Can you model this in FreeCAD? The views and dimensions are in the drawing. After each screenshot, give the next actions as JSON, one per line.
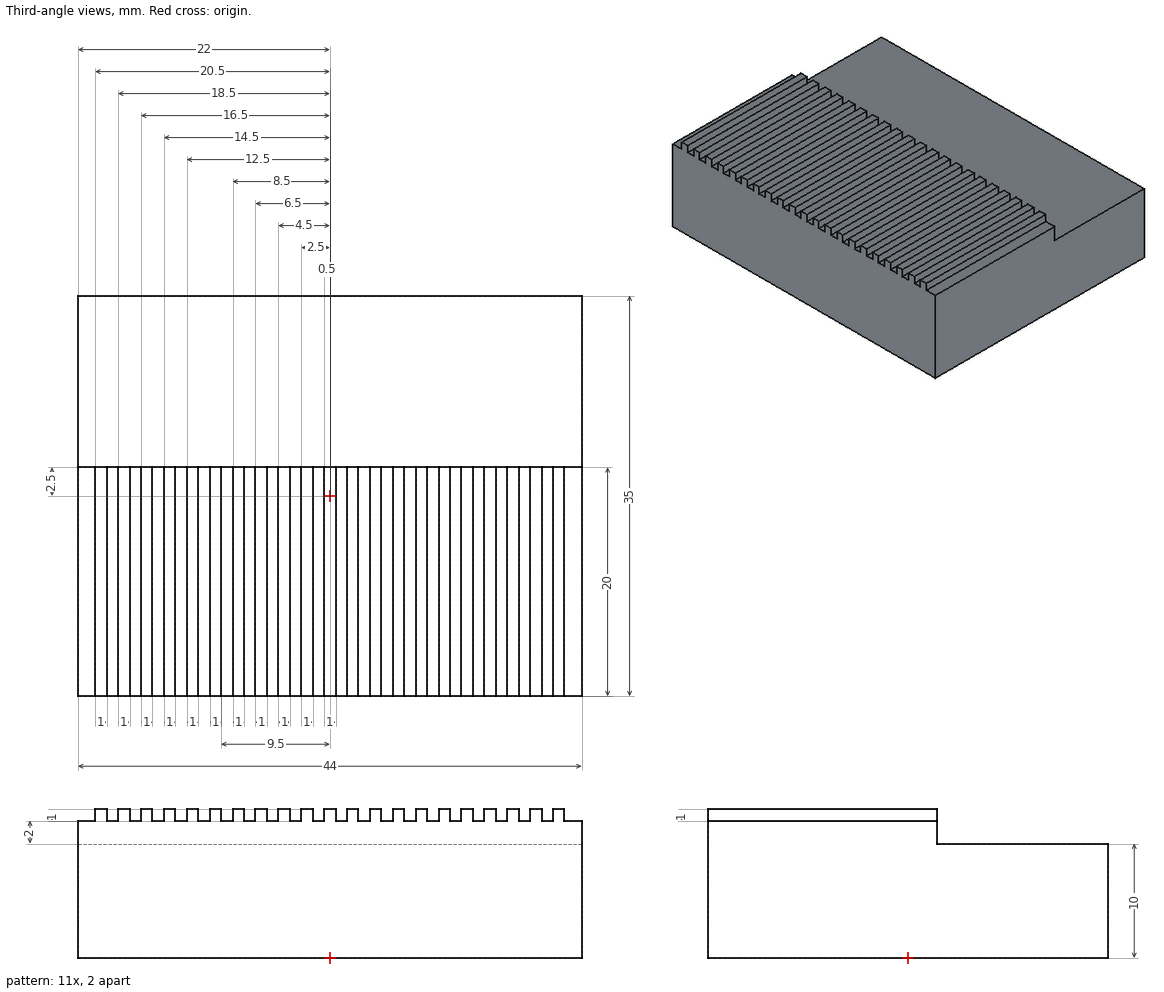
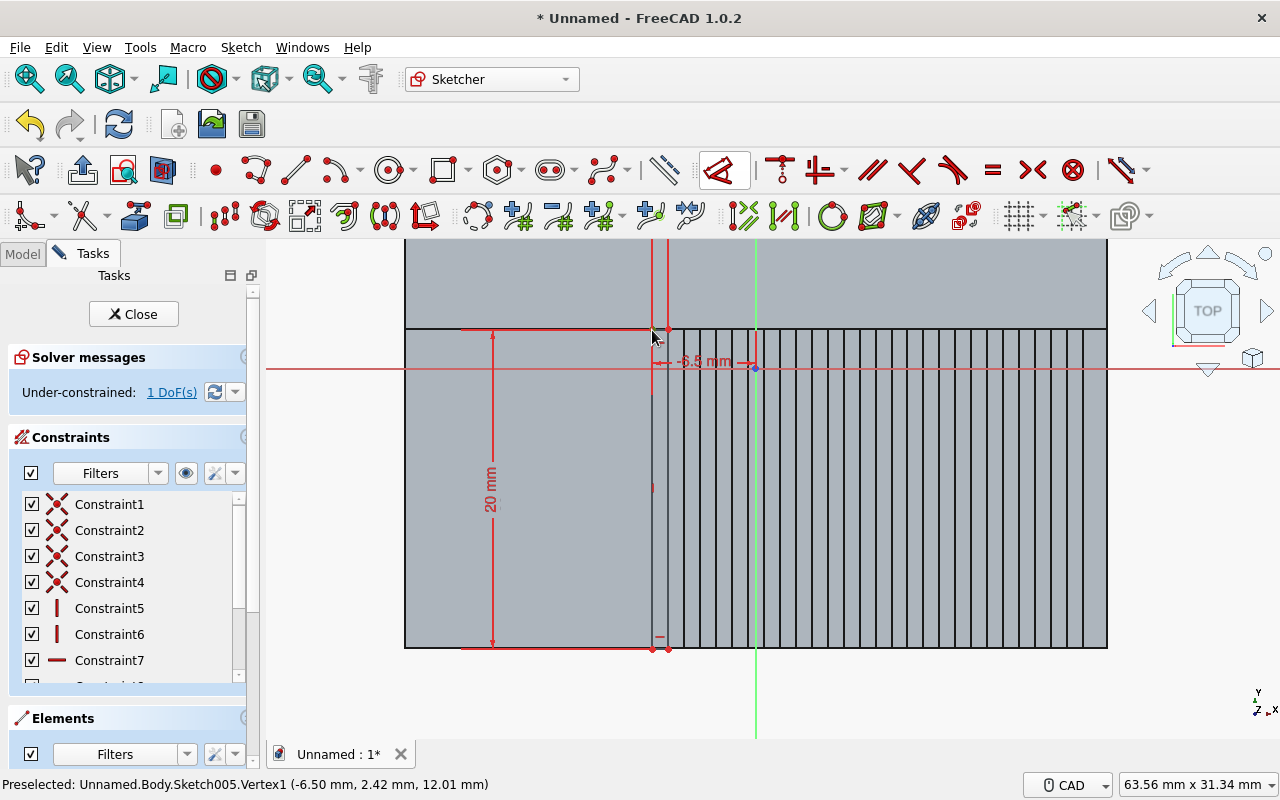
{"action": "left_click", "coordinate": [744, 170]}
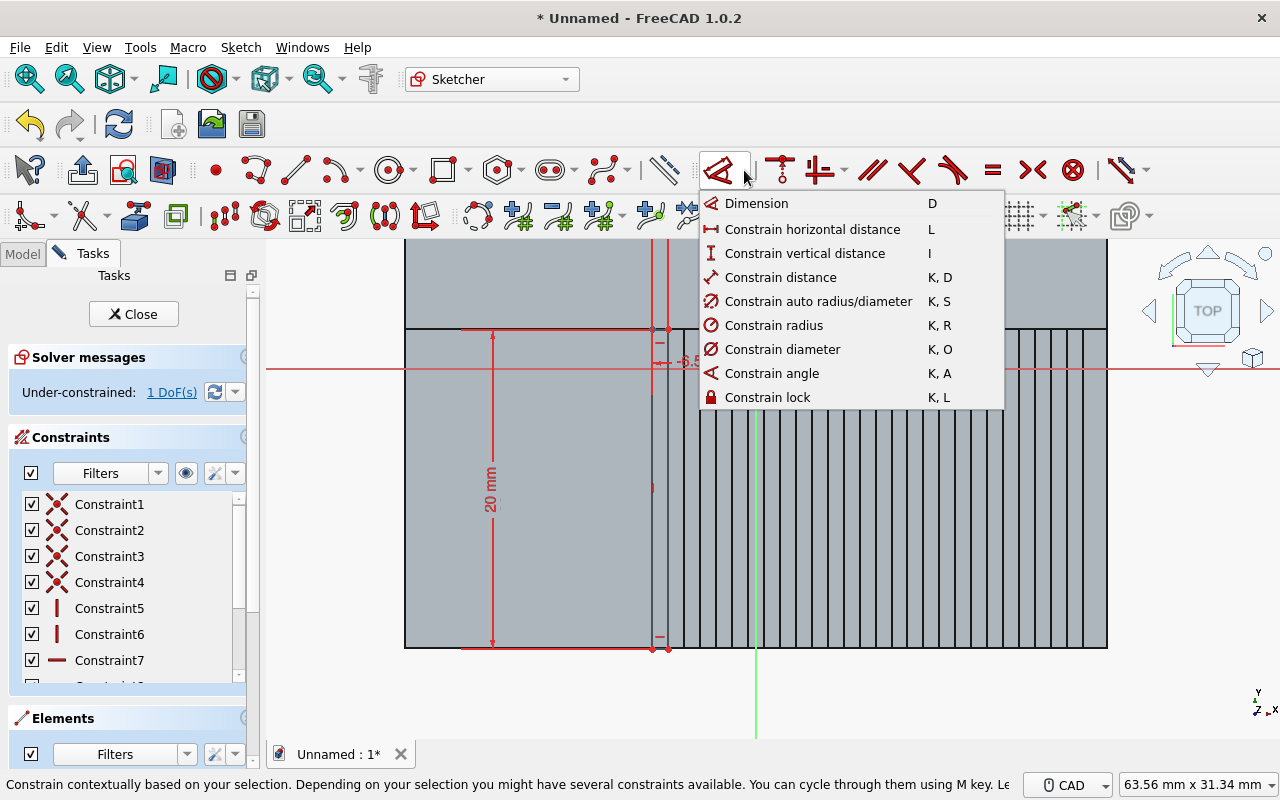
{"action": "left_click", "coordinate": [852, 253]}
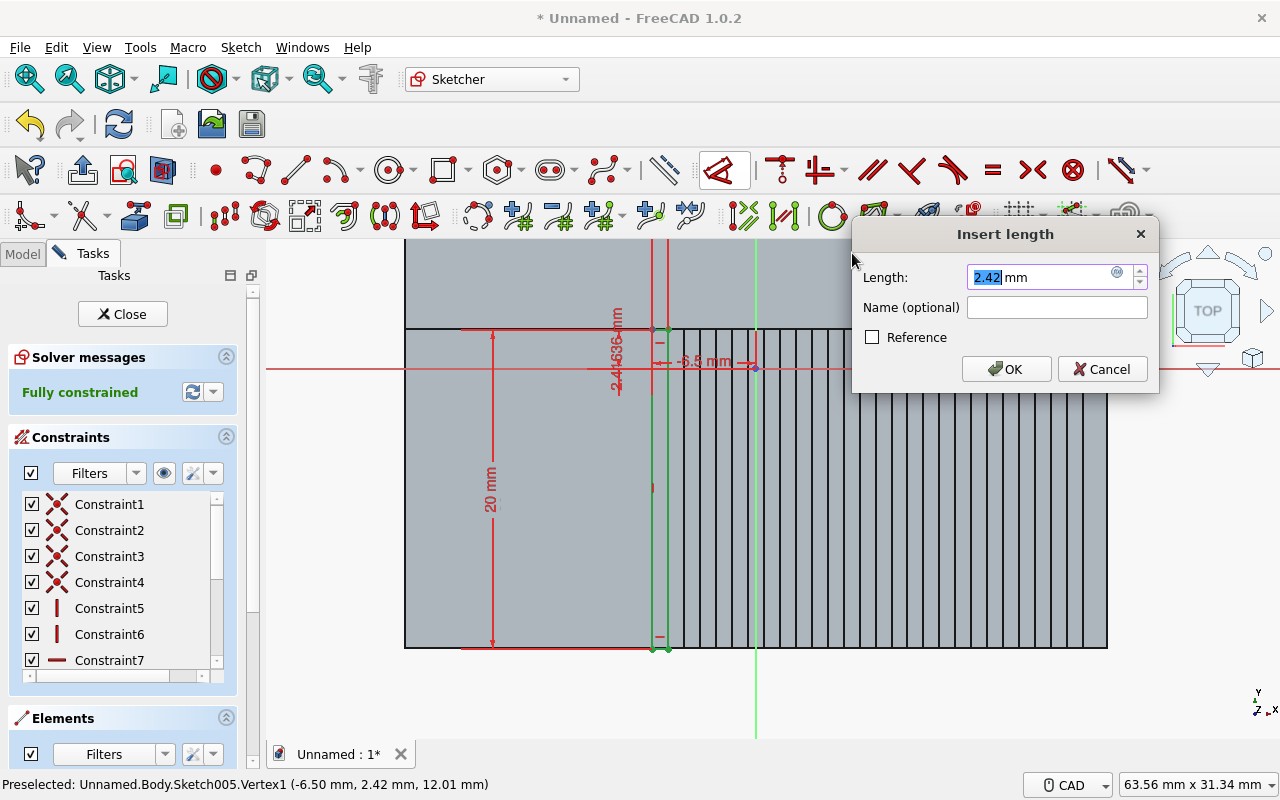
{"action": "type", "text": "2.5"}
{"action": "key", "text": "Return"}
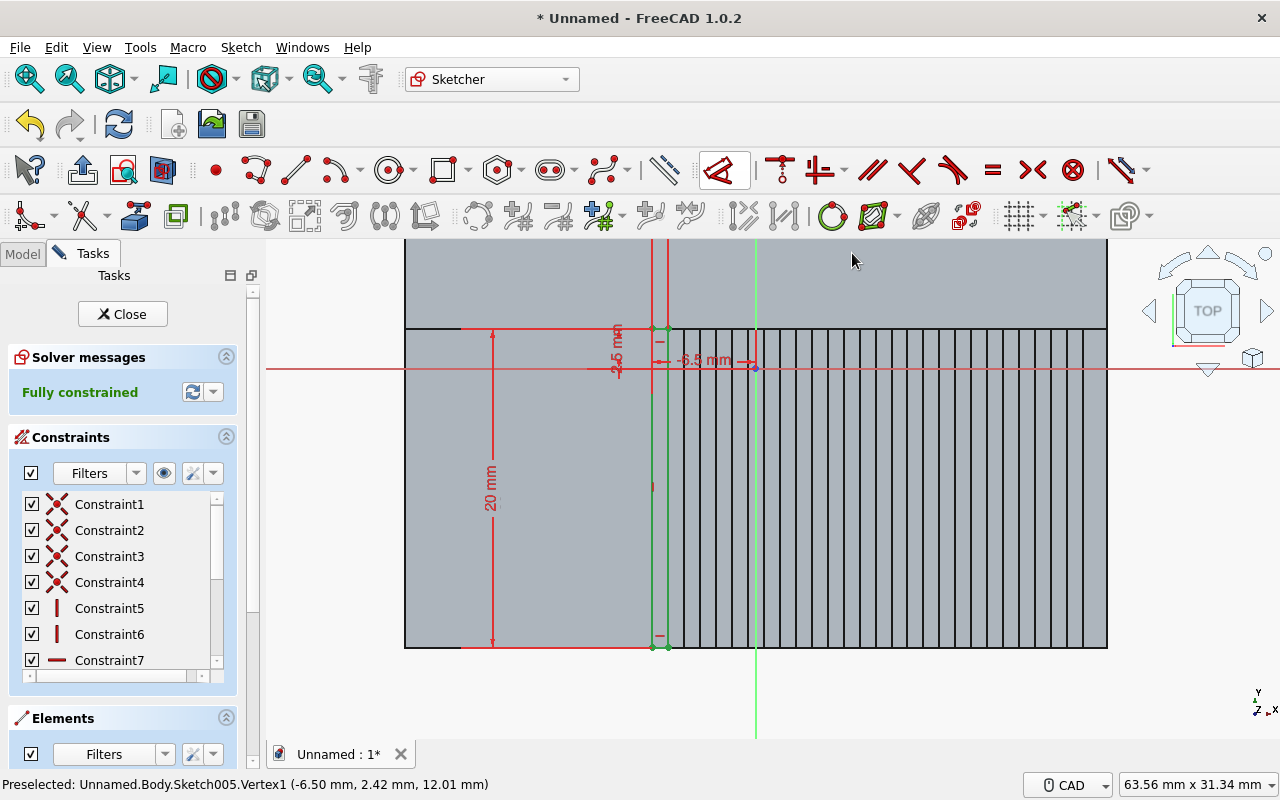
{"action": "left_click", "coordinate": [123, 314]}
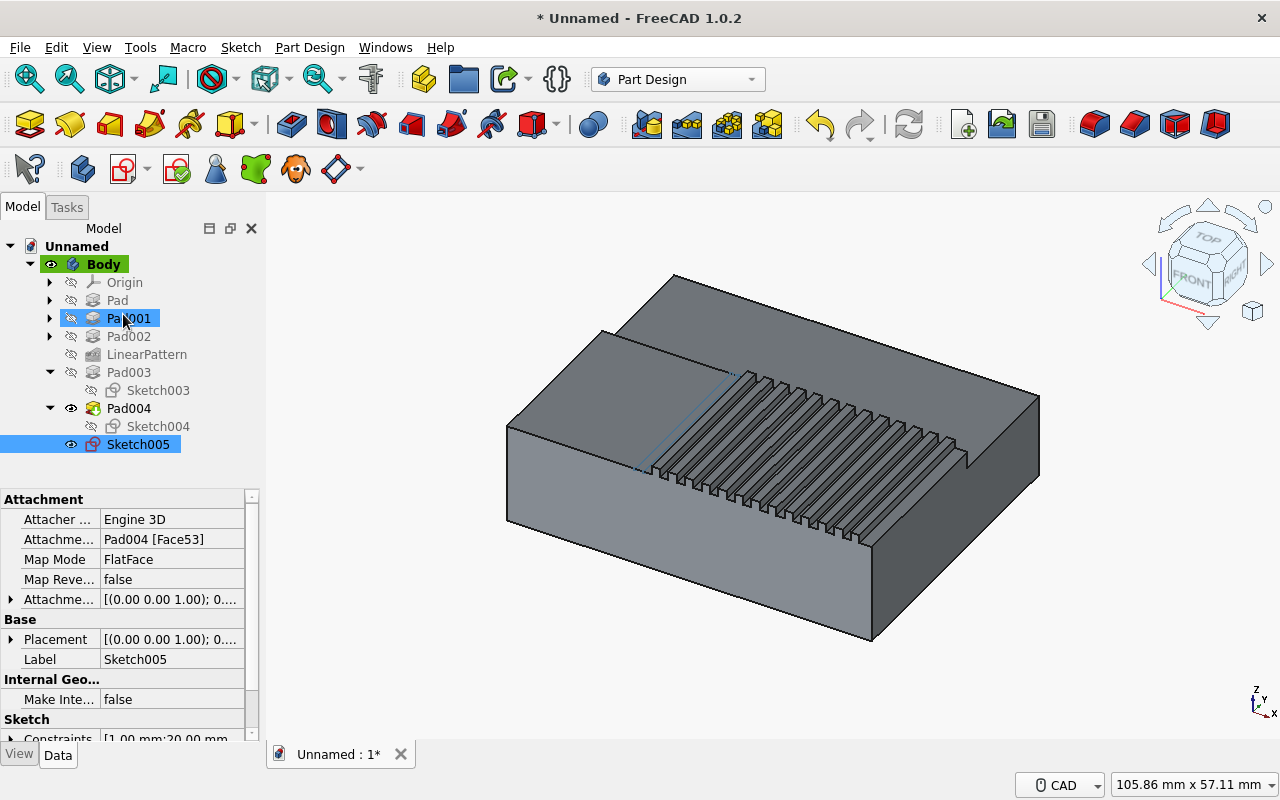
{"action": "left_click", "coordinate": [30, 124]}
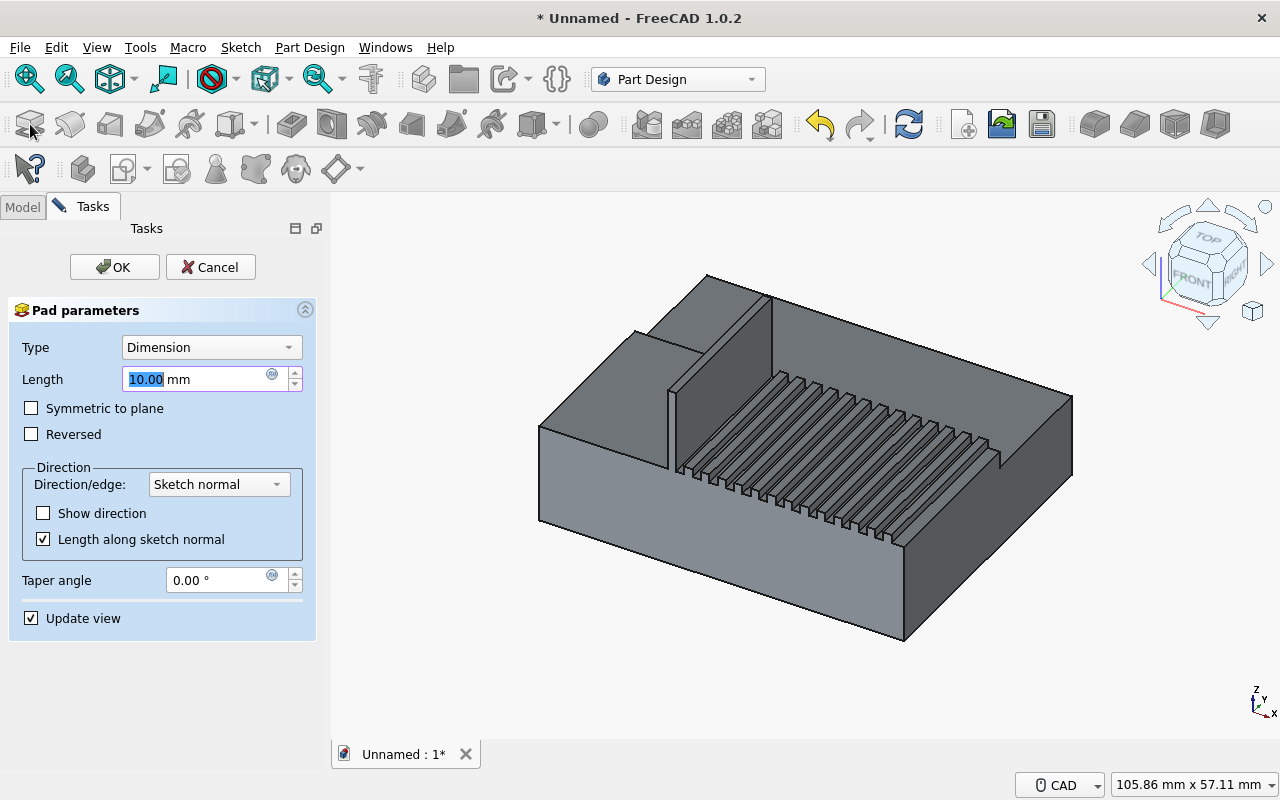
{"action": "type", "text": "1"}
{"action": "key", "text": "Tab"}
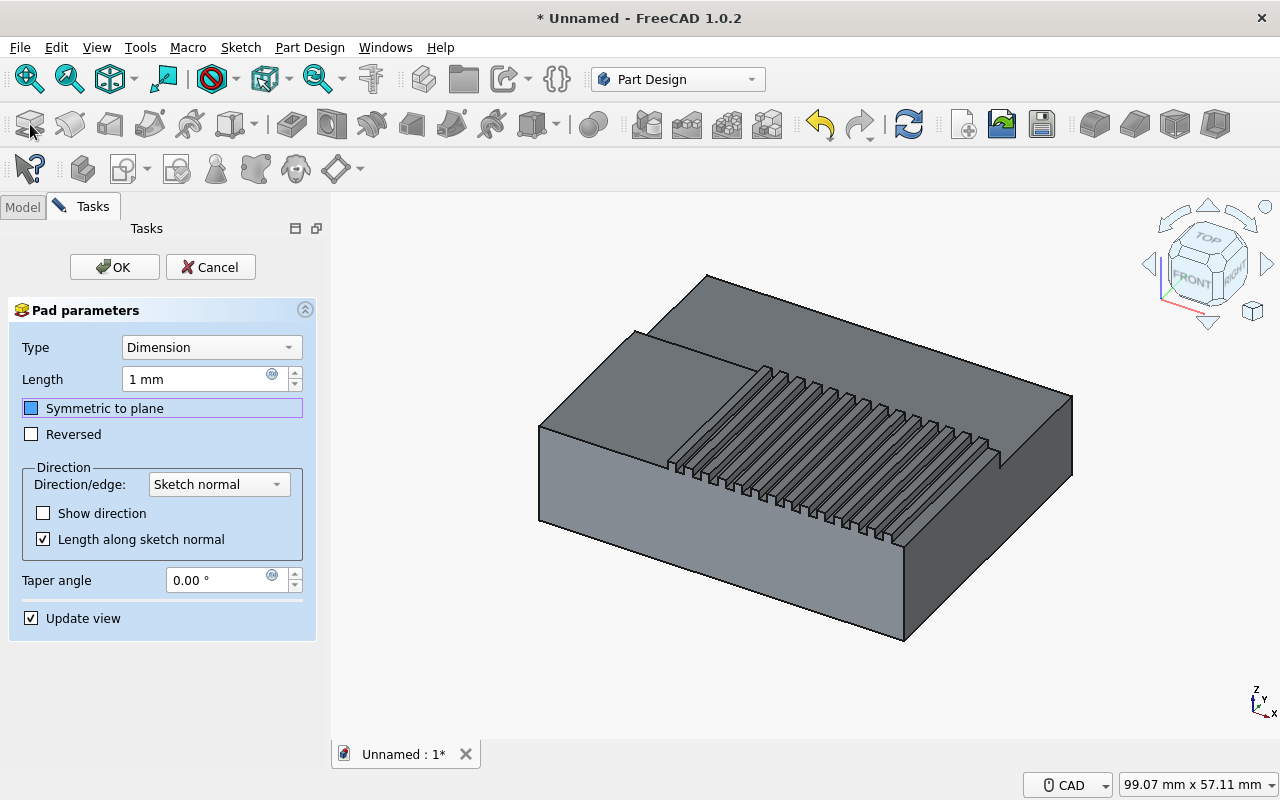
{"action": "left_click", "coordinate": [115, 267]}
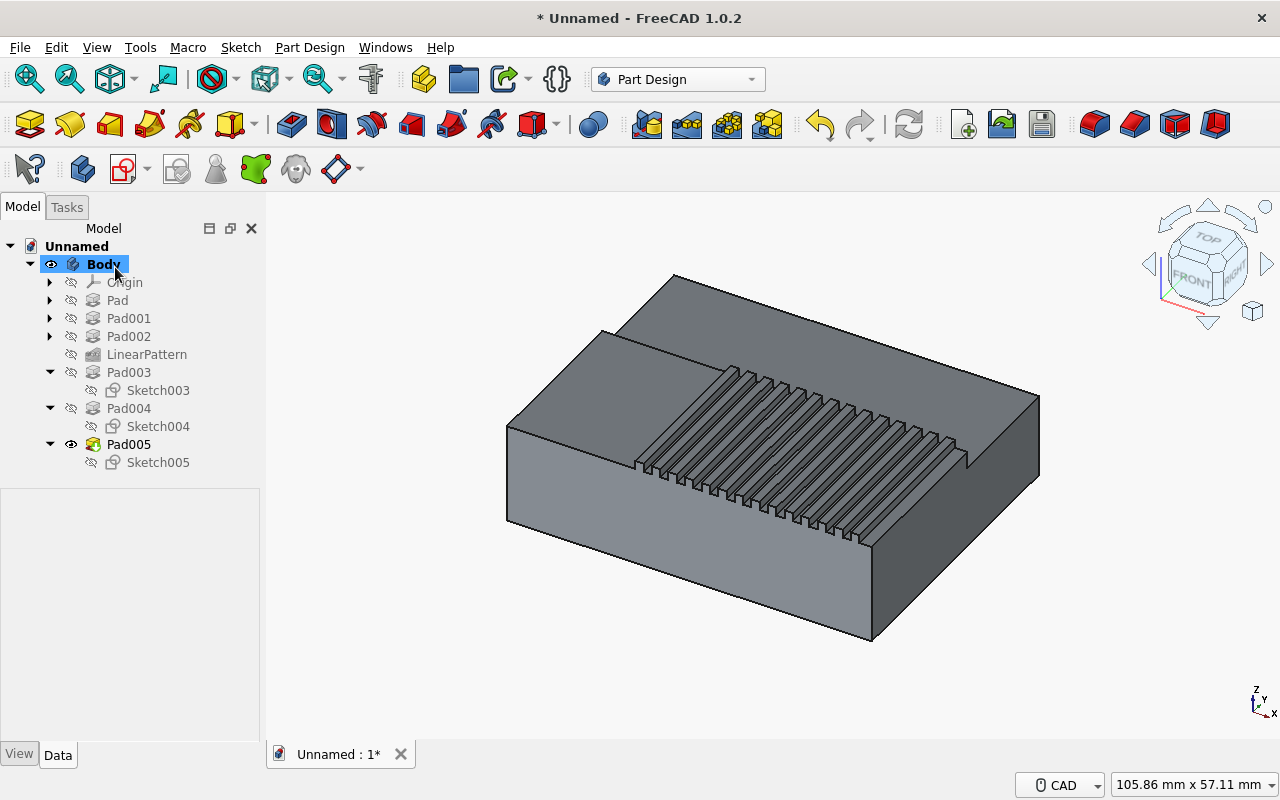
{"action": "left_click", "coordinate": [619, 399]}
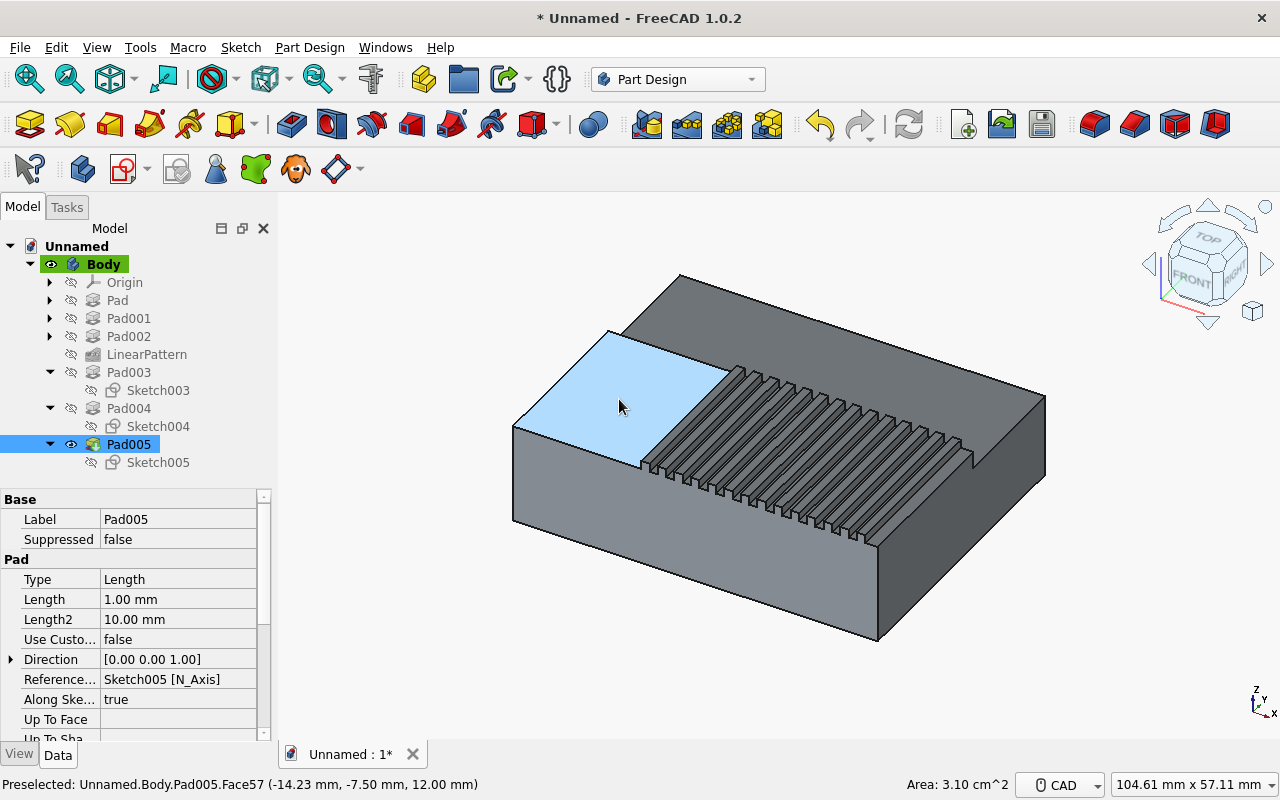
{"action": "left_click", "coordinate": [124, 170]}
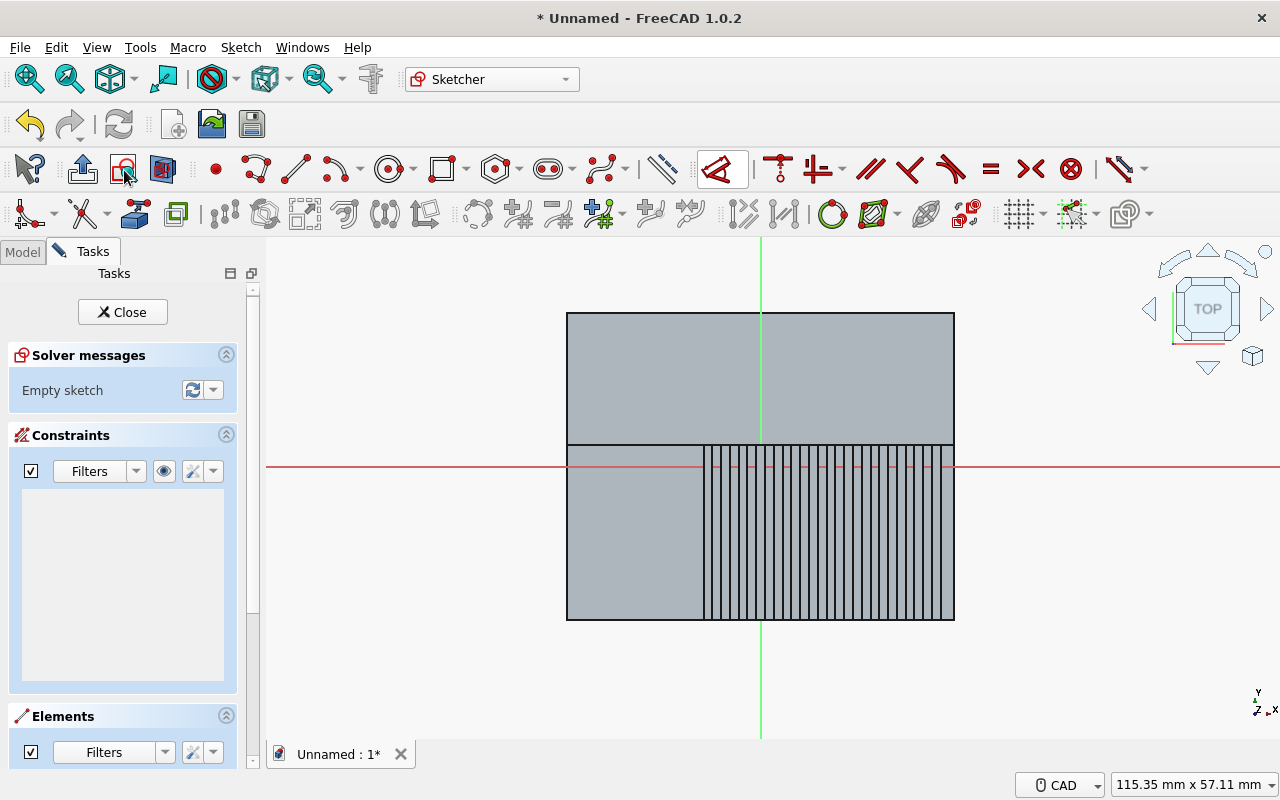
{"action": "left_click", "coordinate": [164, 170]}